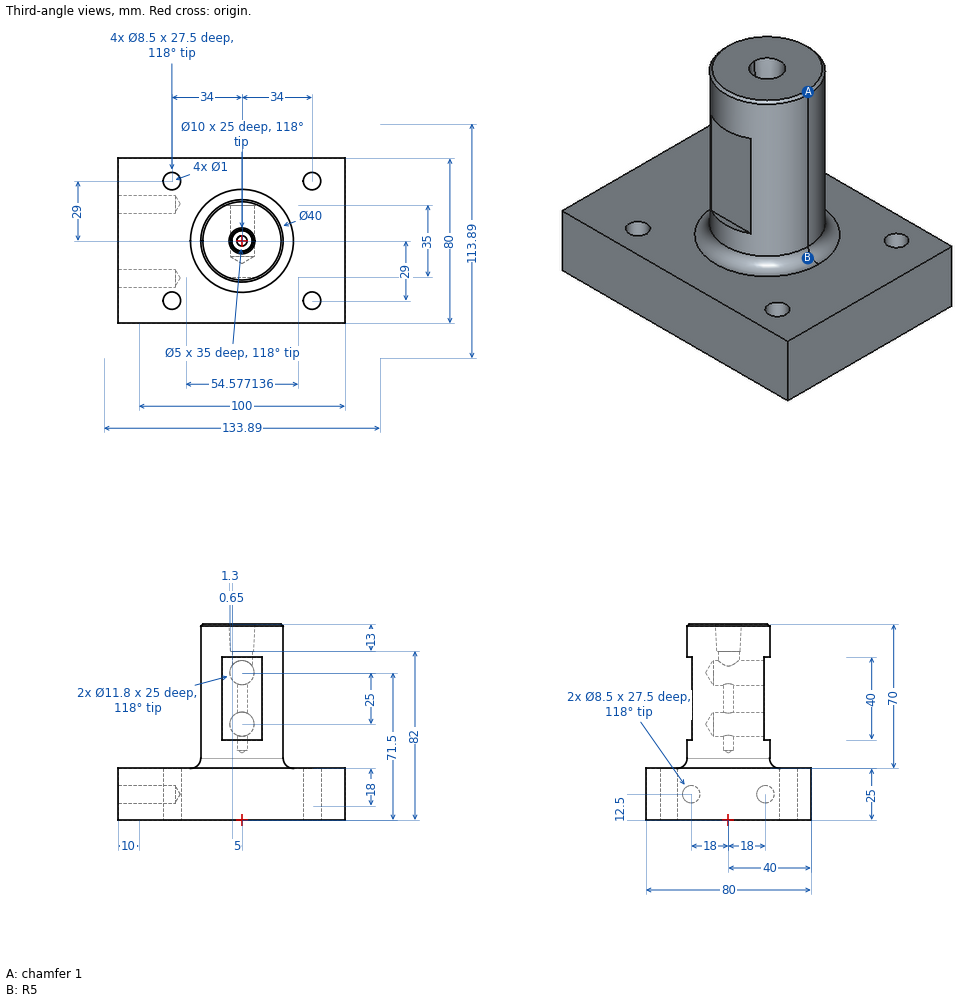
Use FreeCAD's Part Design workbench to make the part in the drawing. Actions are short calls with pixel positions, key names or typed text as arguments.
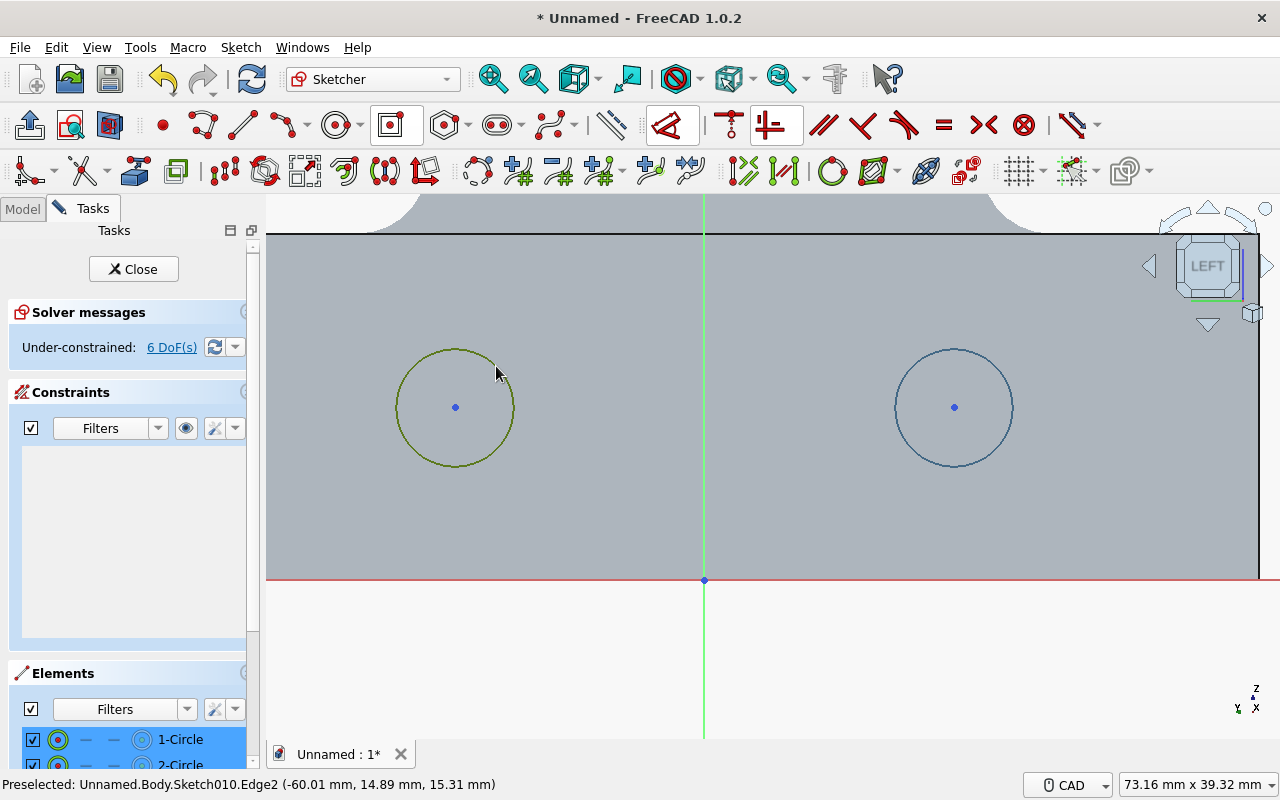
click(944, 126)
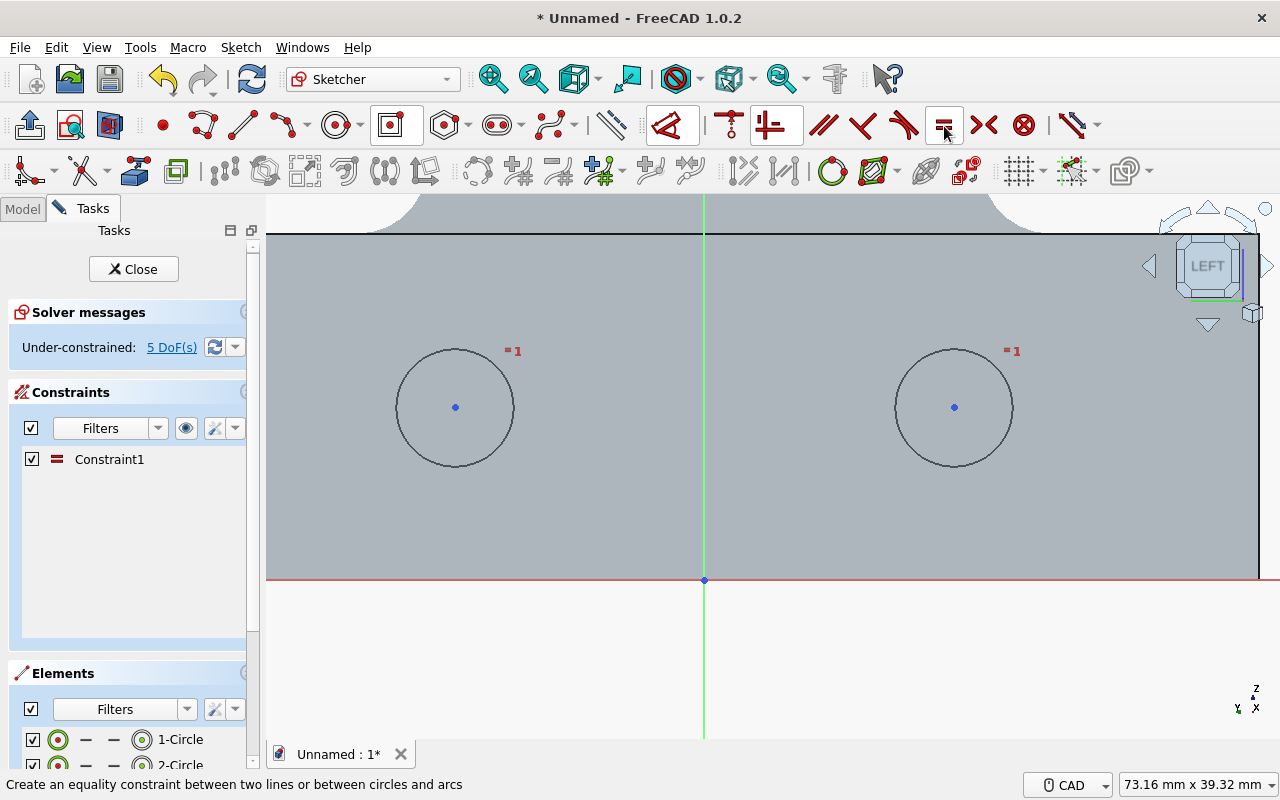
click(995, 366)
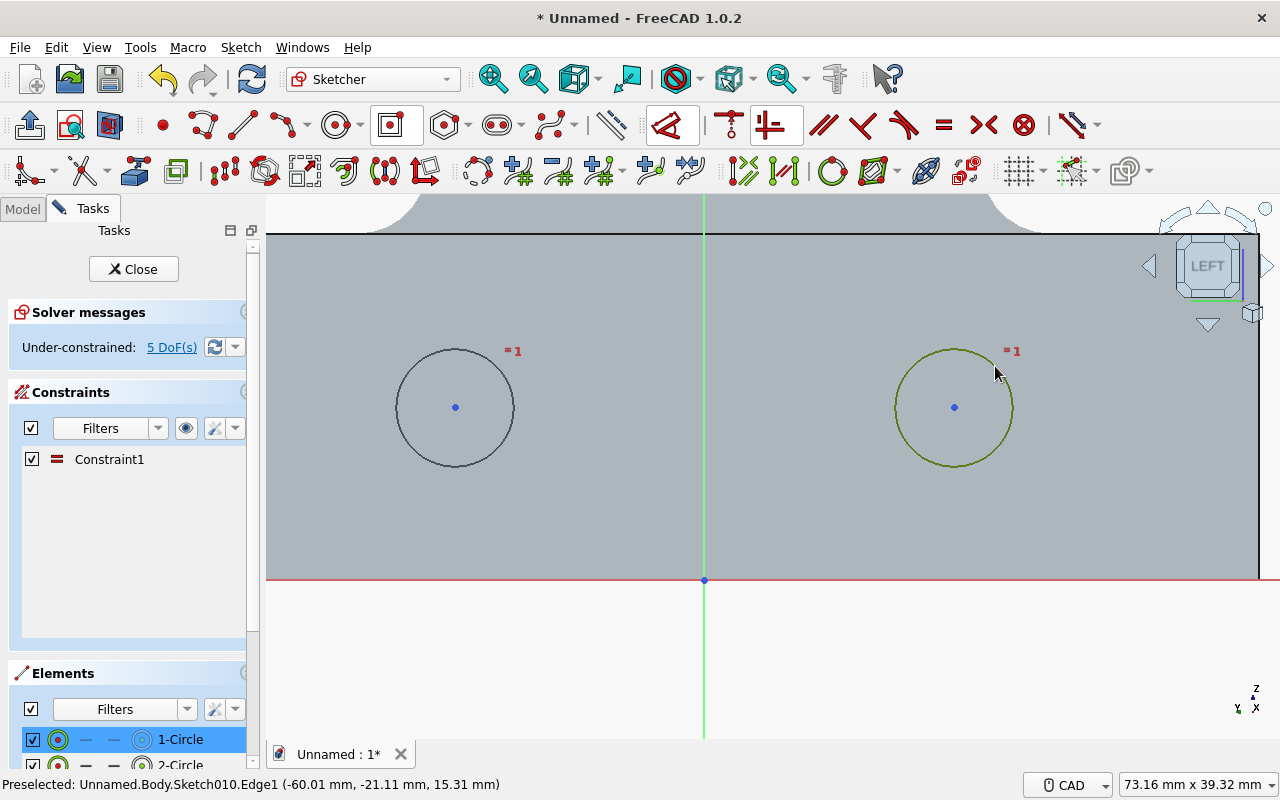
key(k)
key(o)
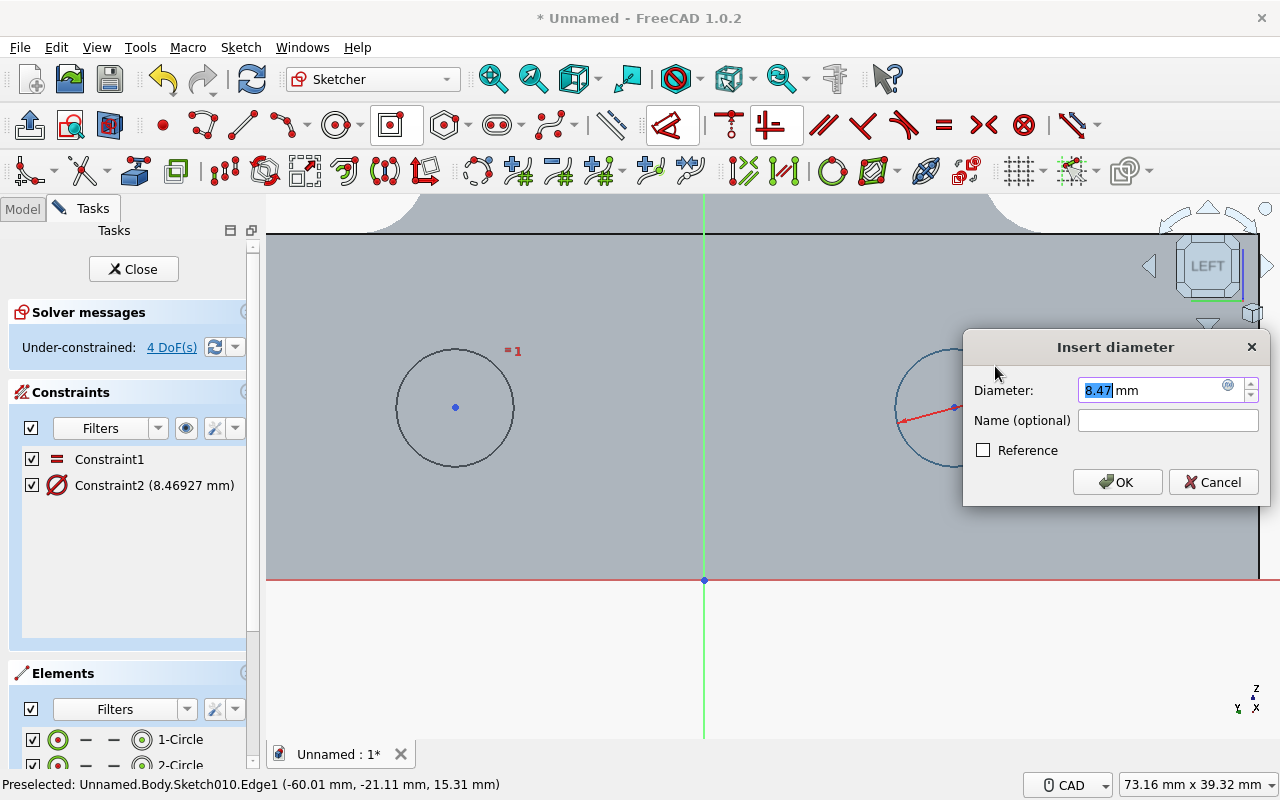
text(8.5)
key(Return)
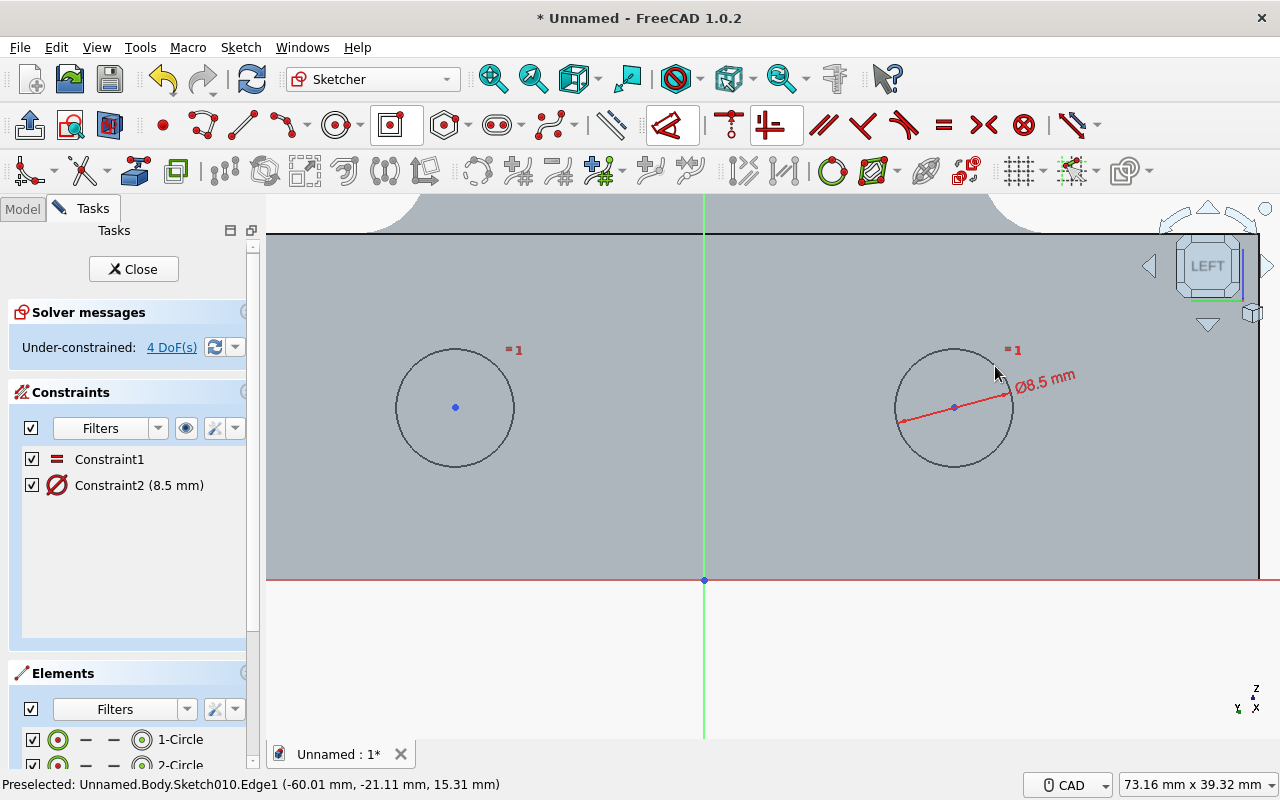
click(954, 408)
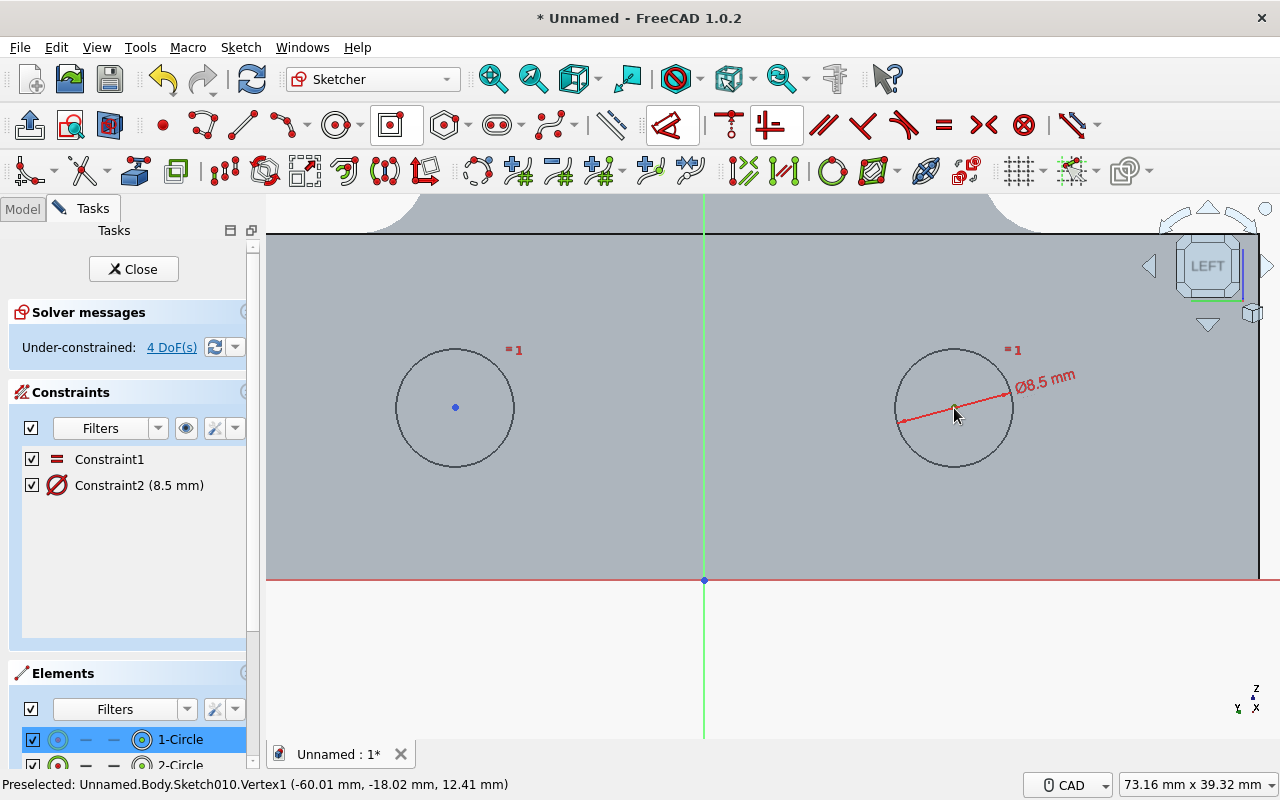
key(l)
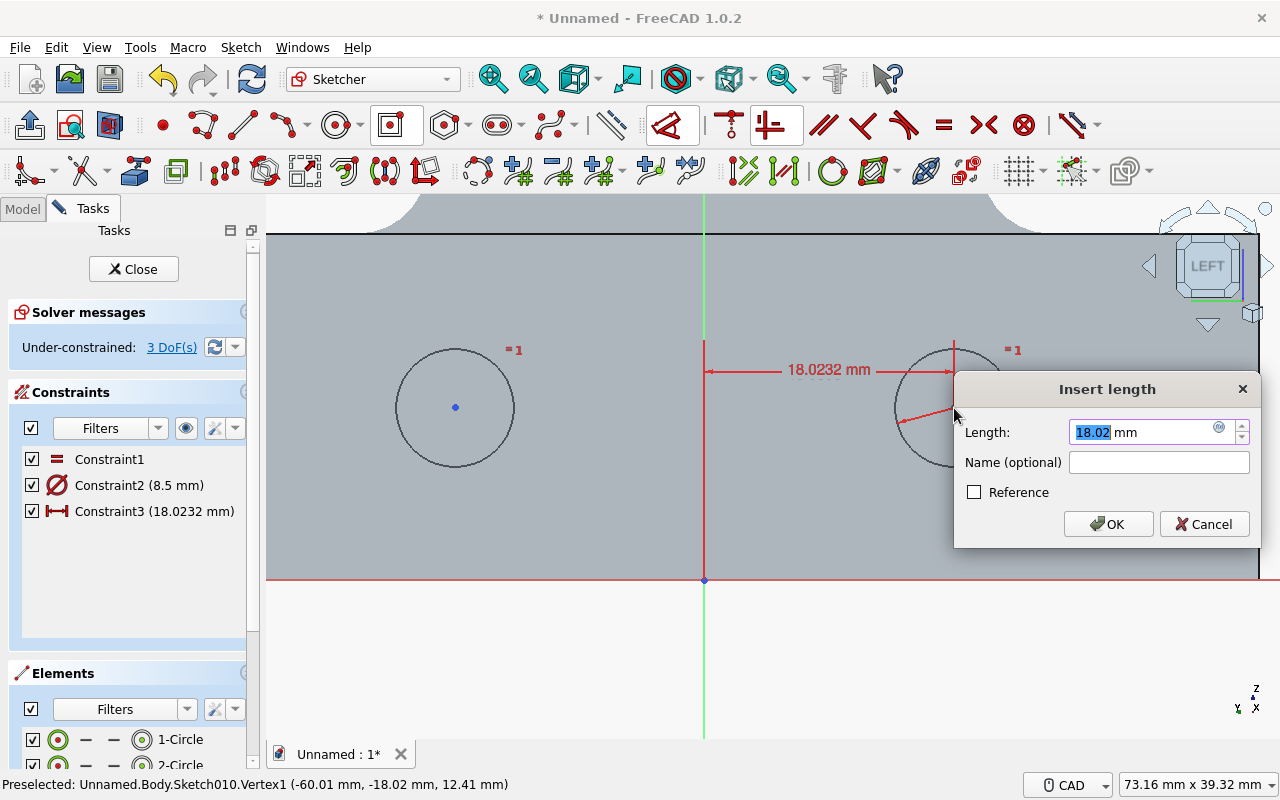
text(18)
key(Return)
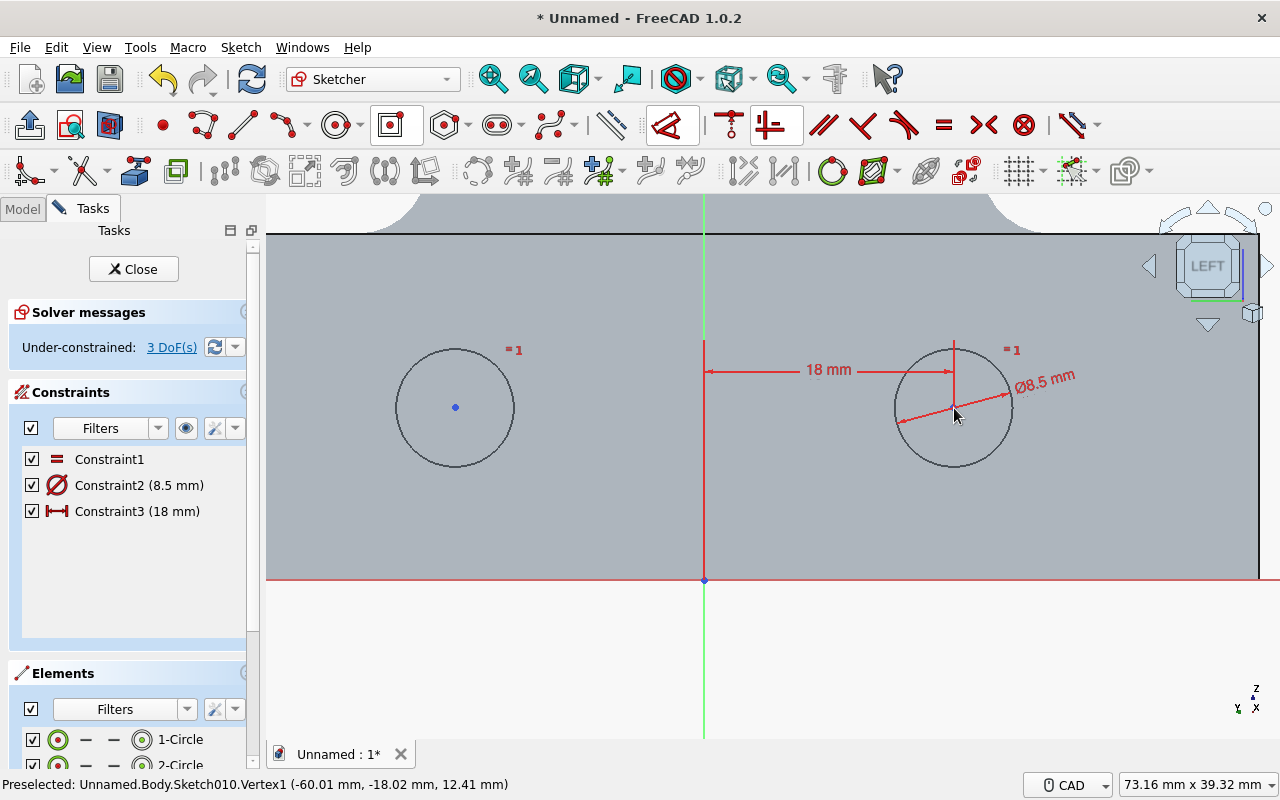
click(455, 408)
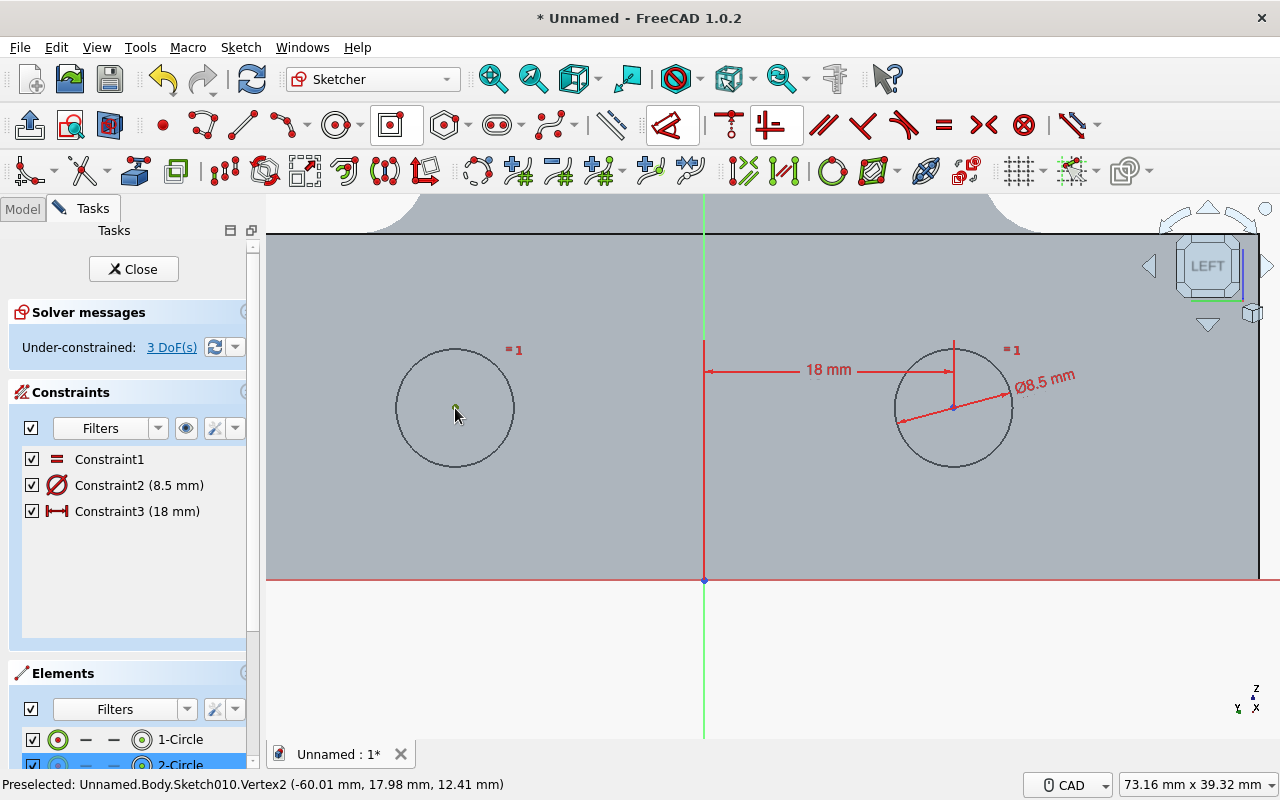
key(l)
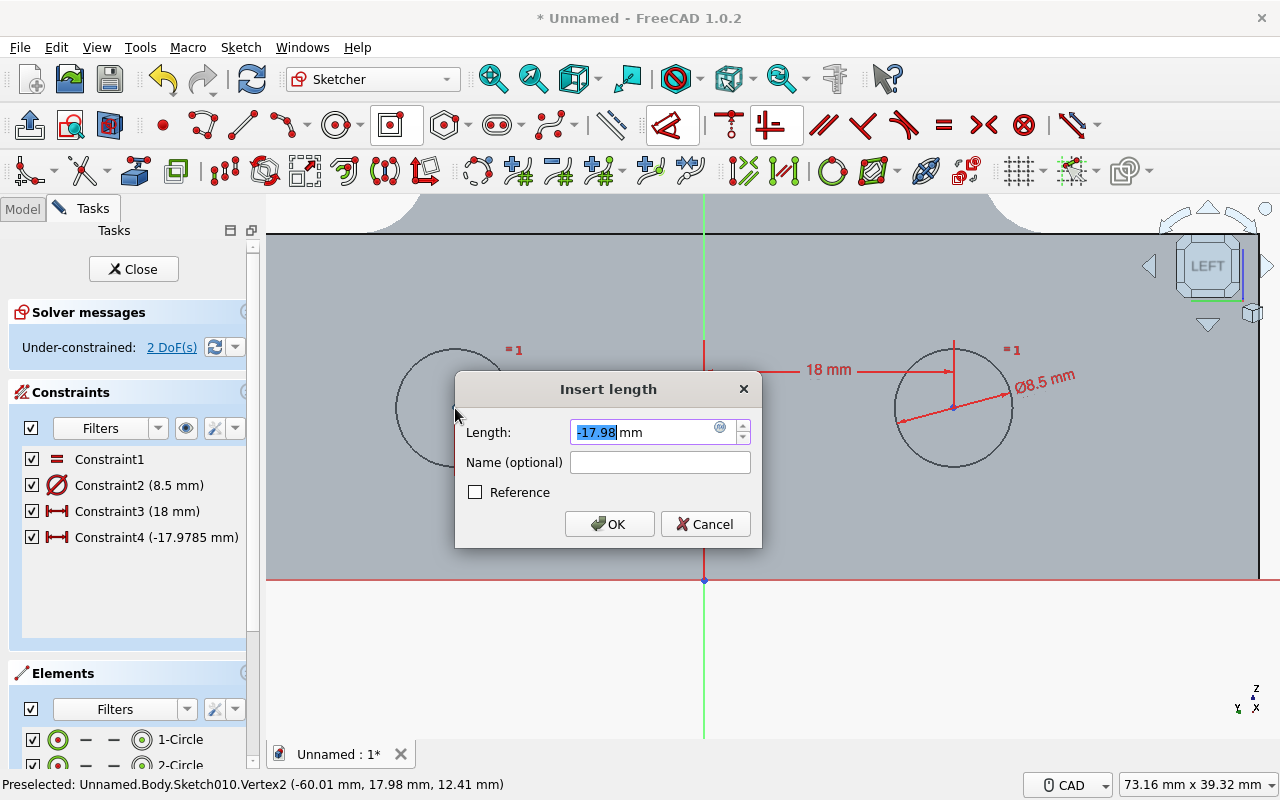
text(-18)
key(Return)